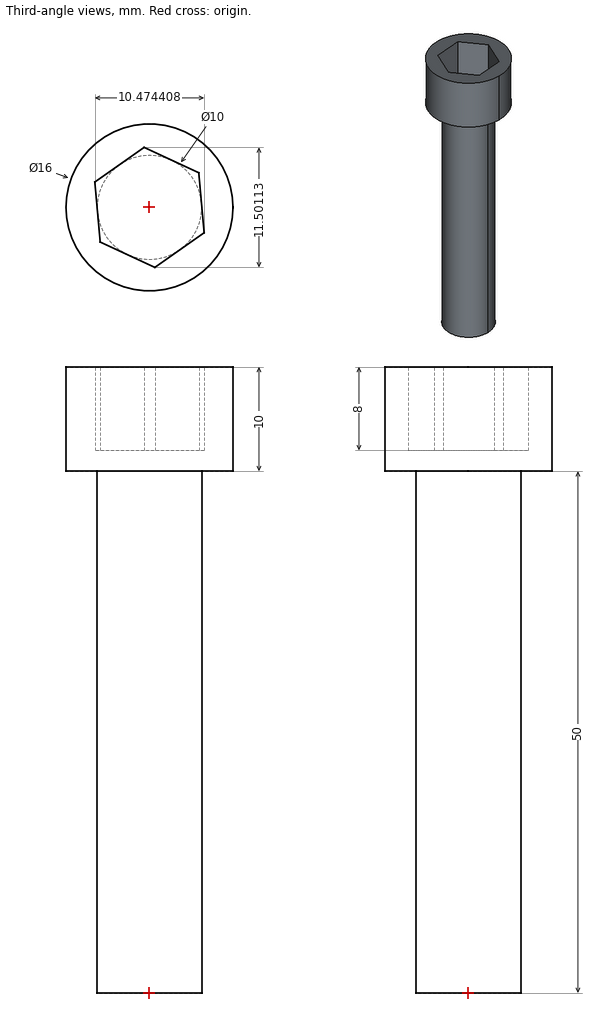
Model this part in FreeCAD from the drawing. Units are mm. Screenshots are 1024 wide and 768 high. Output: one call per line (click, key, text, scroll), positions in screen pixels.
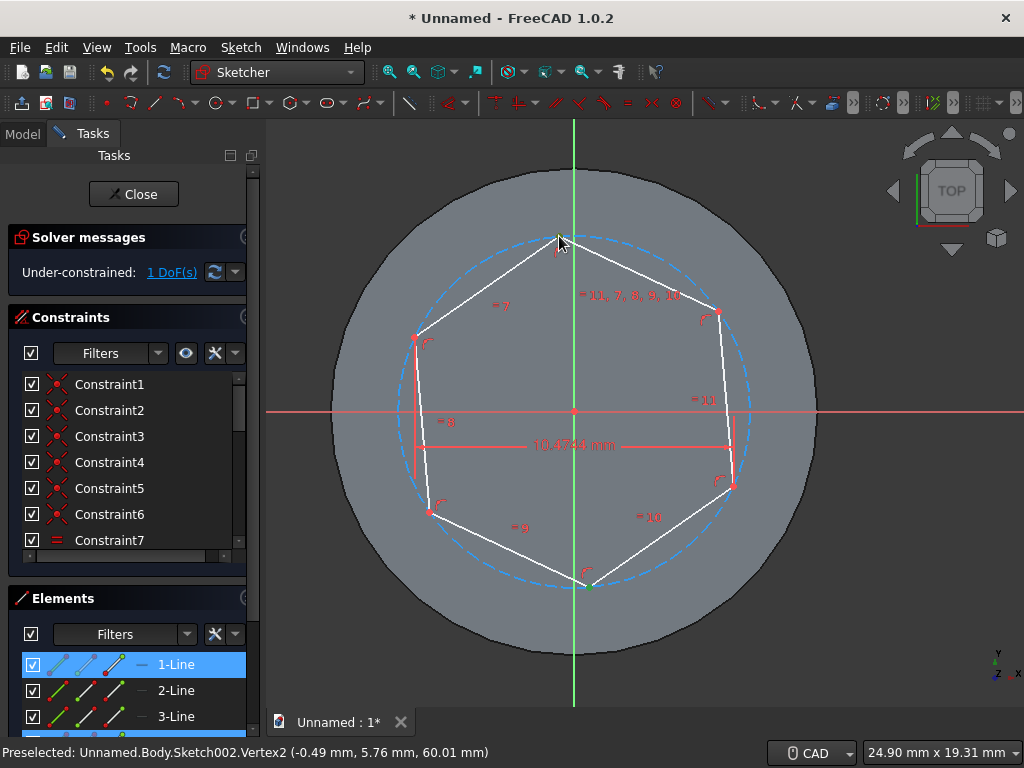
key(i)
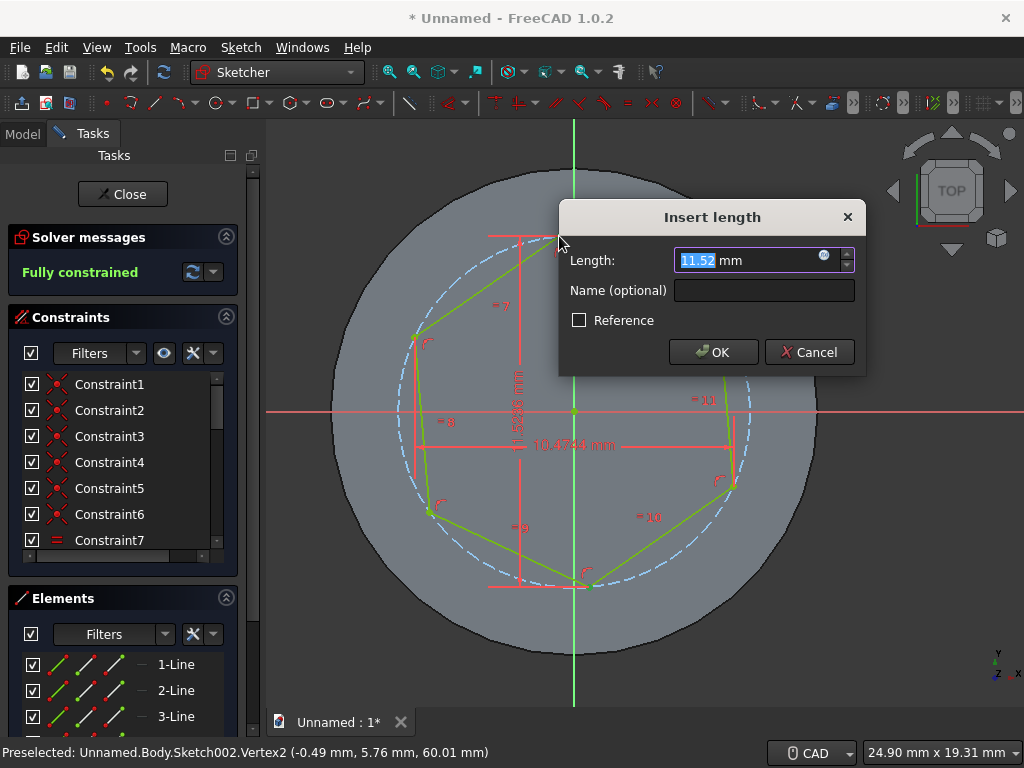
text(11.50113)
key(Return)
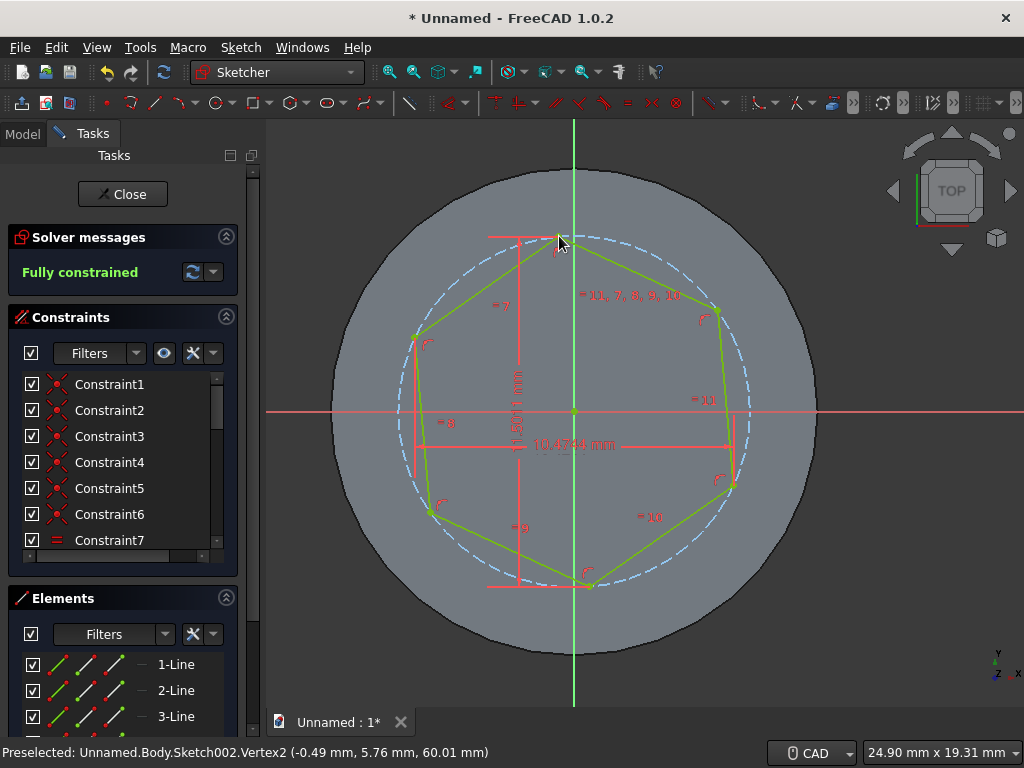
click(123, 194)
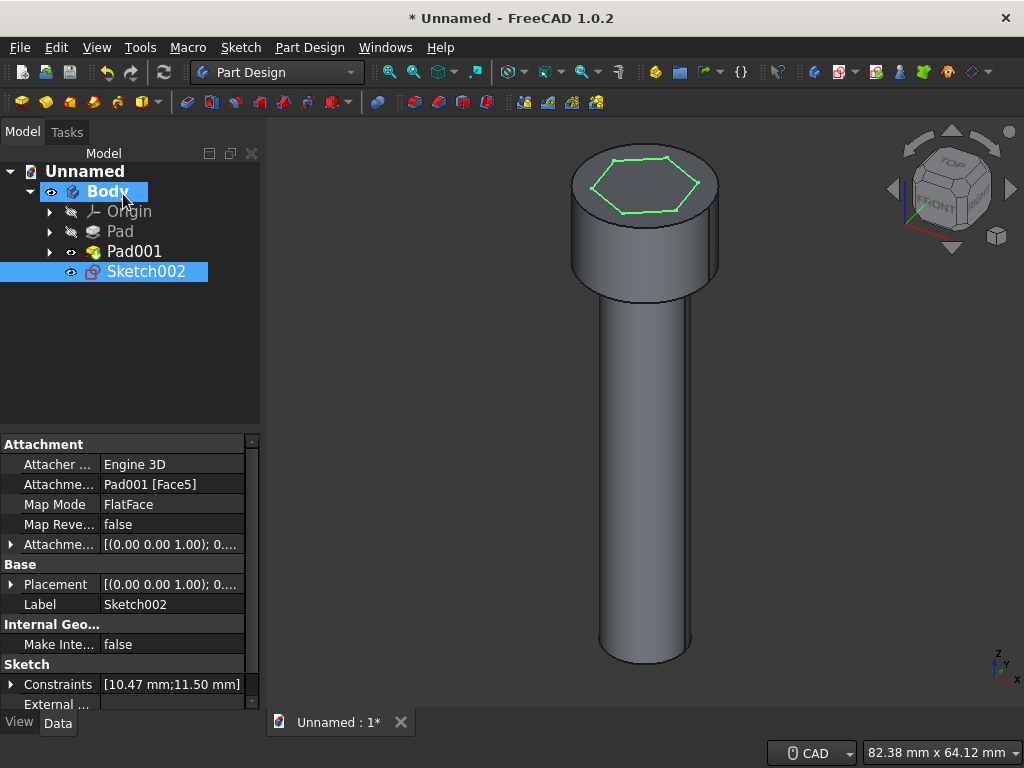
click(188, 102)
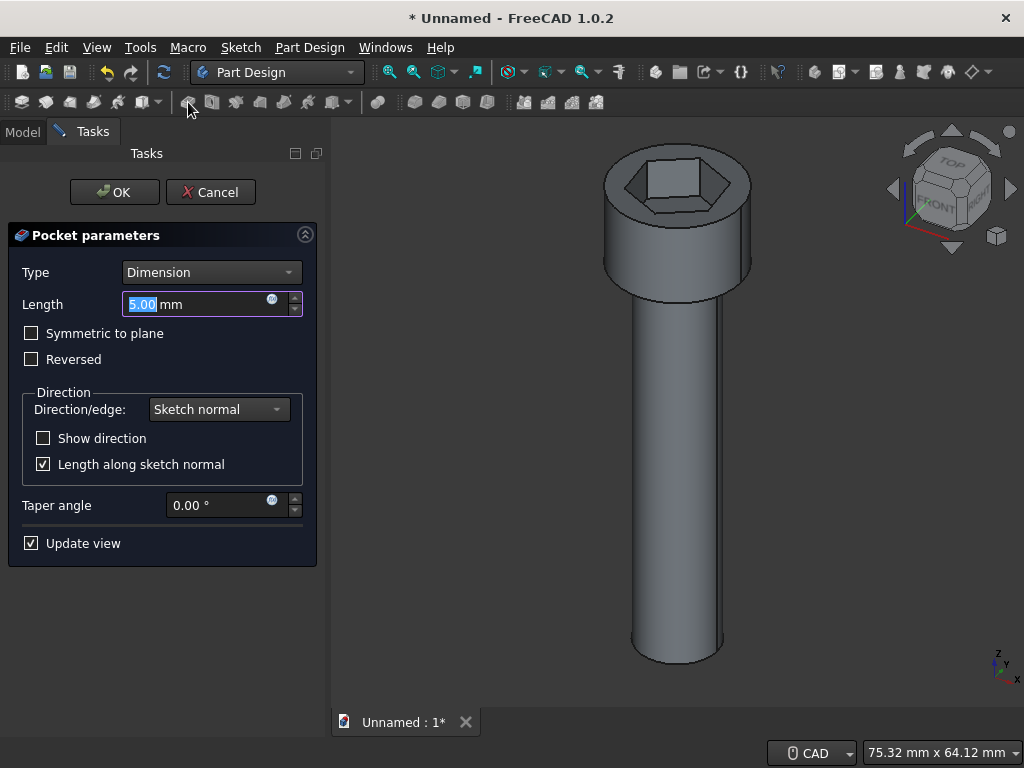
text(8)
key(Tab)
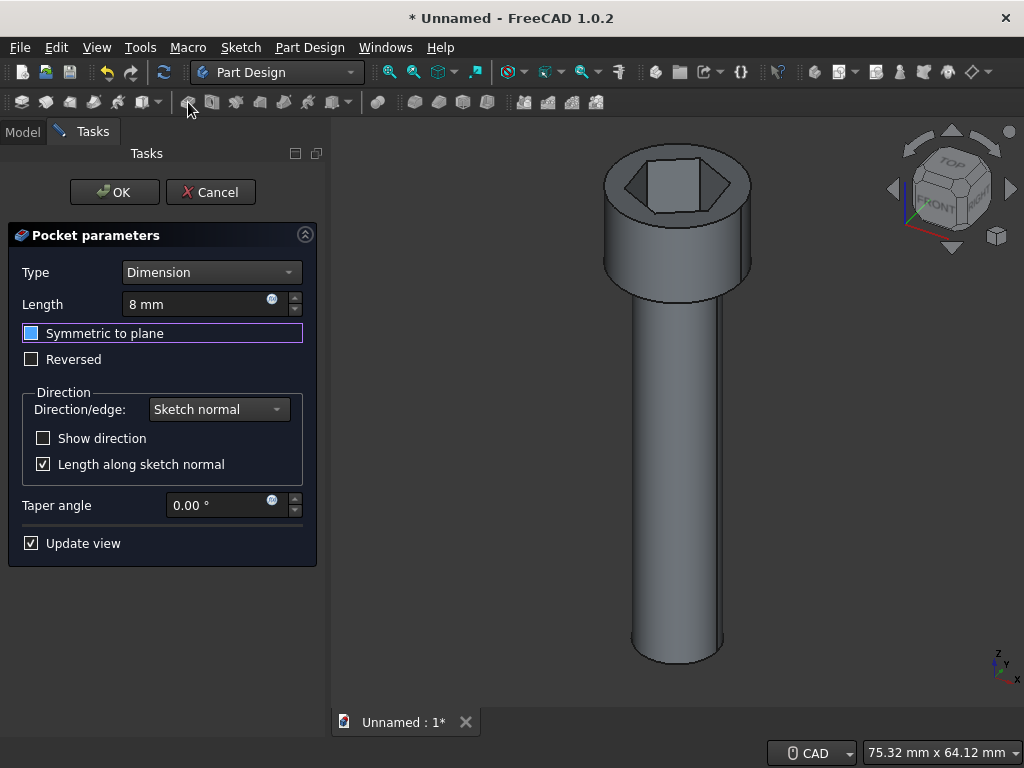
click(115, 192)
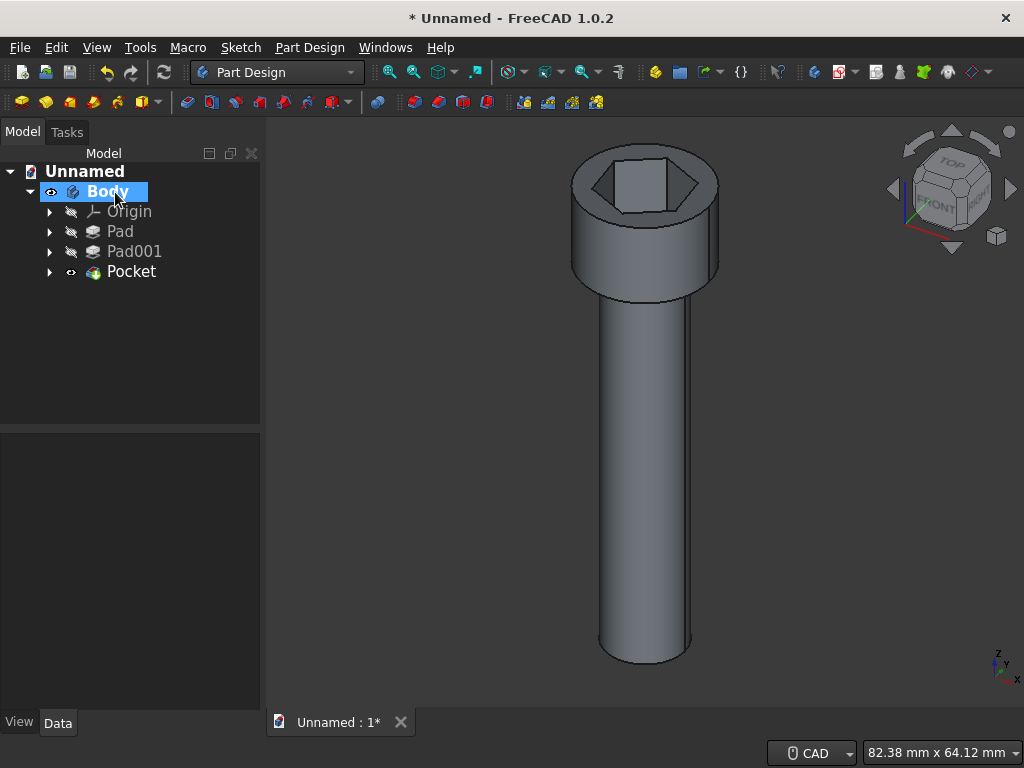
key(0)